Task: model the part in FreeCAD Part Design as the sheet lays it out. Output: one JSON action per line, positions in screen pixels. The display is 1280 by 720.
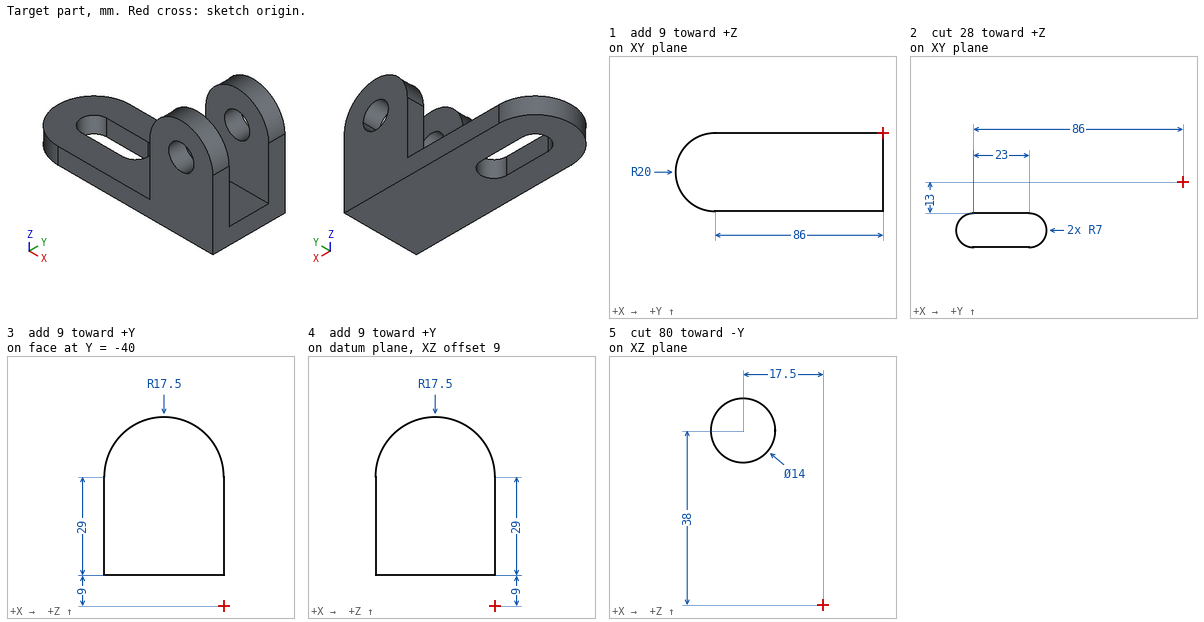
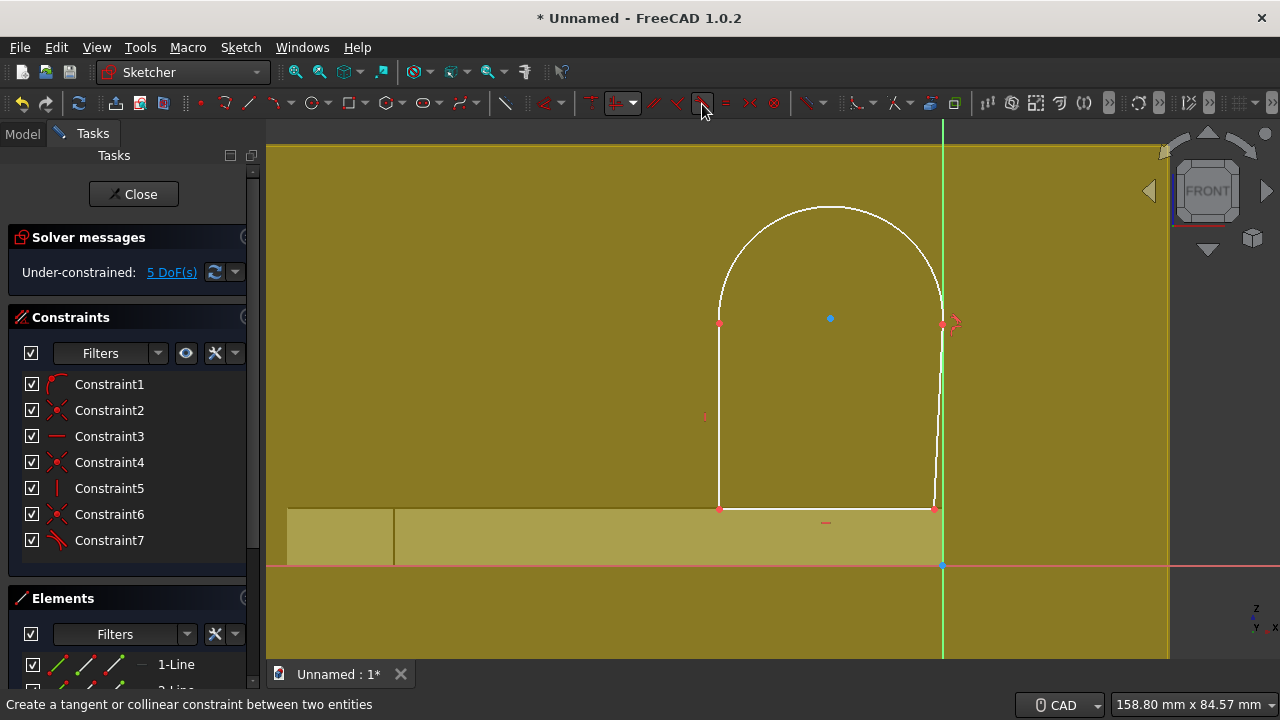
{"action": "left_click", "coordinate": [719, 454]}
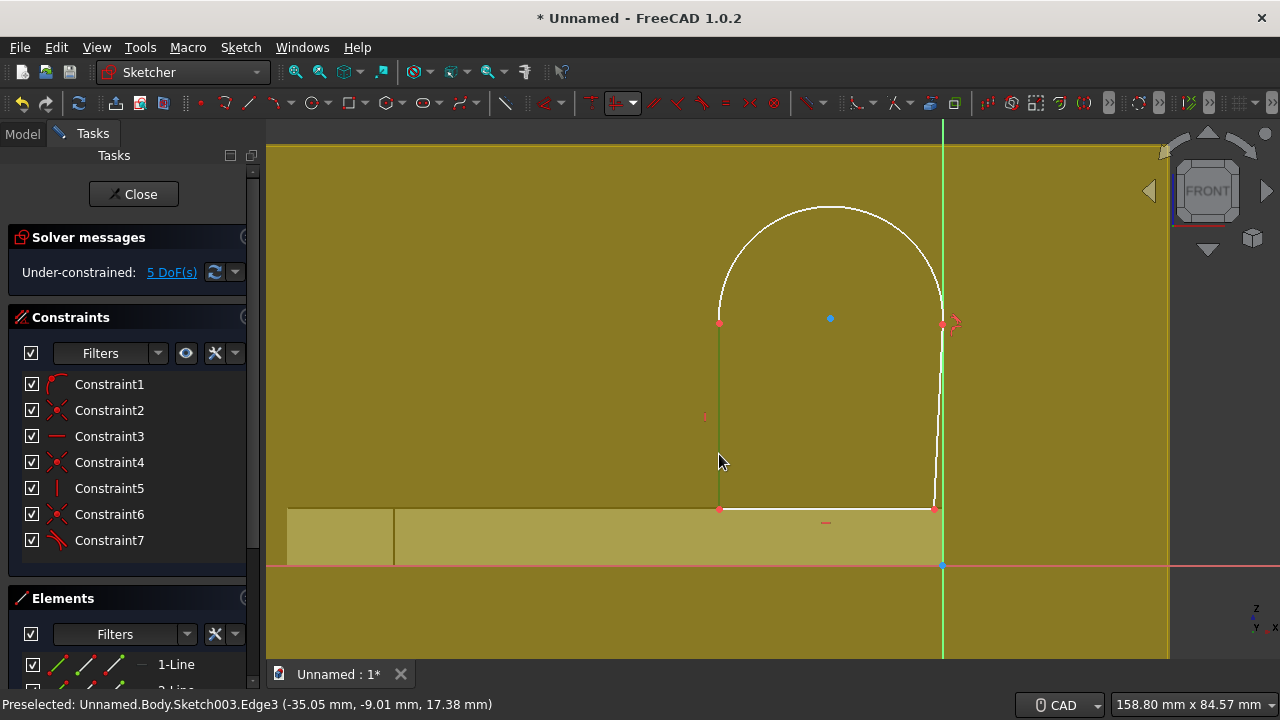
{"action": "left_click", "coordinate": [898, 229]}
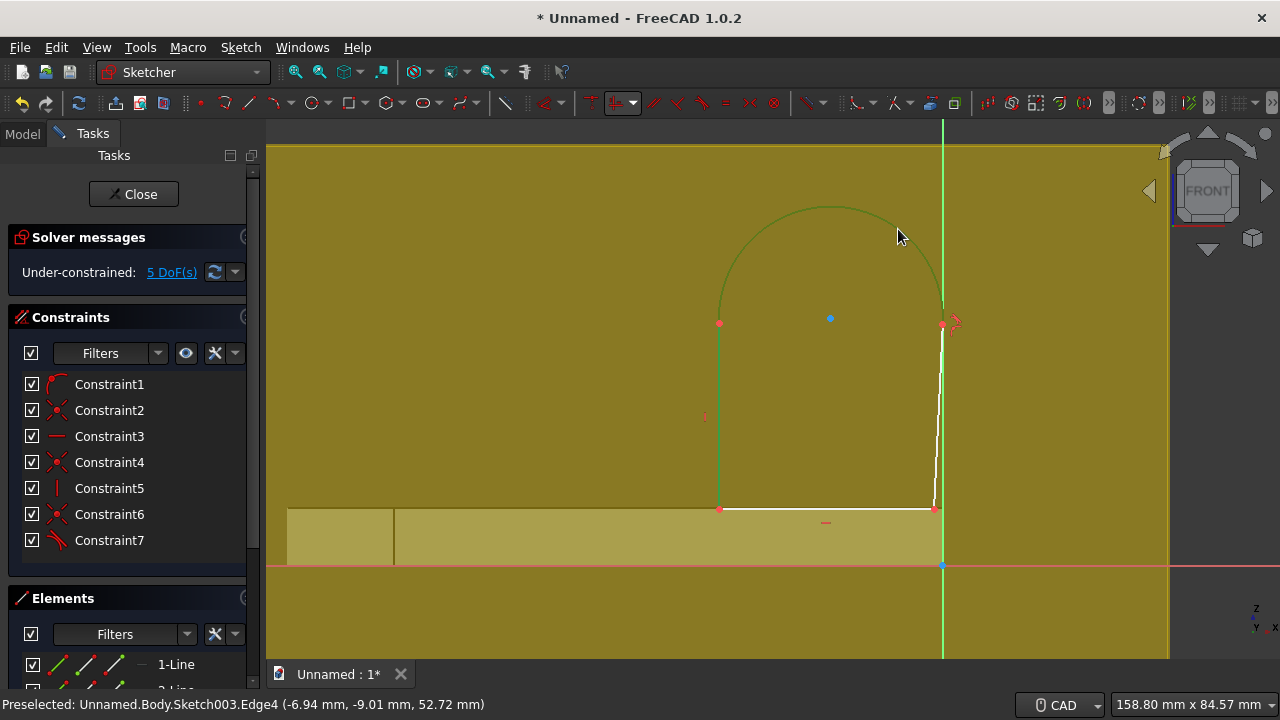
{"action": "left_click", "coordinate": [702, 104]}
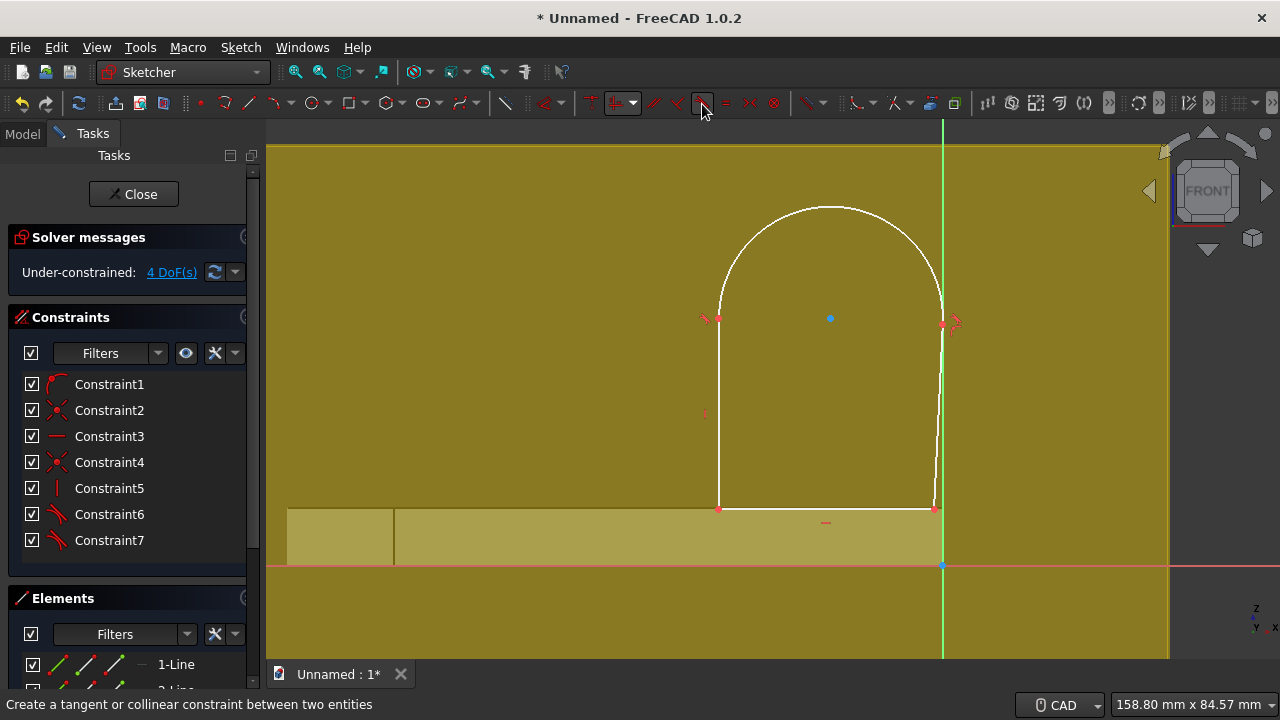
{"action": "left_click", "coordinate": [940, 380]}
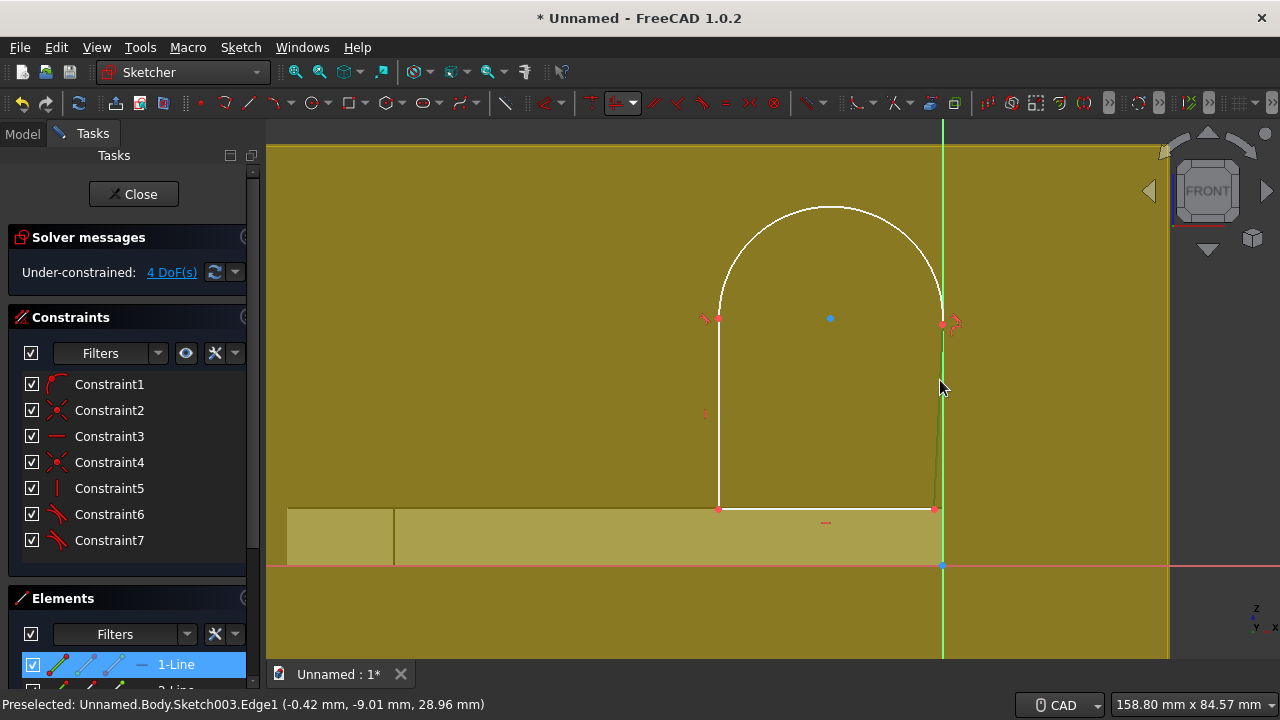
{"action": "left_click", "coordinate": [636, 104]}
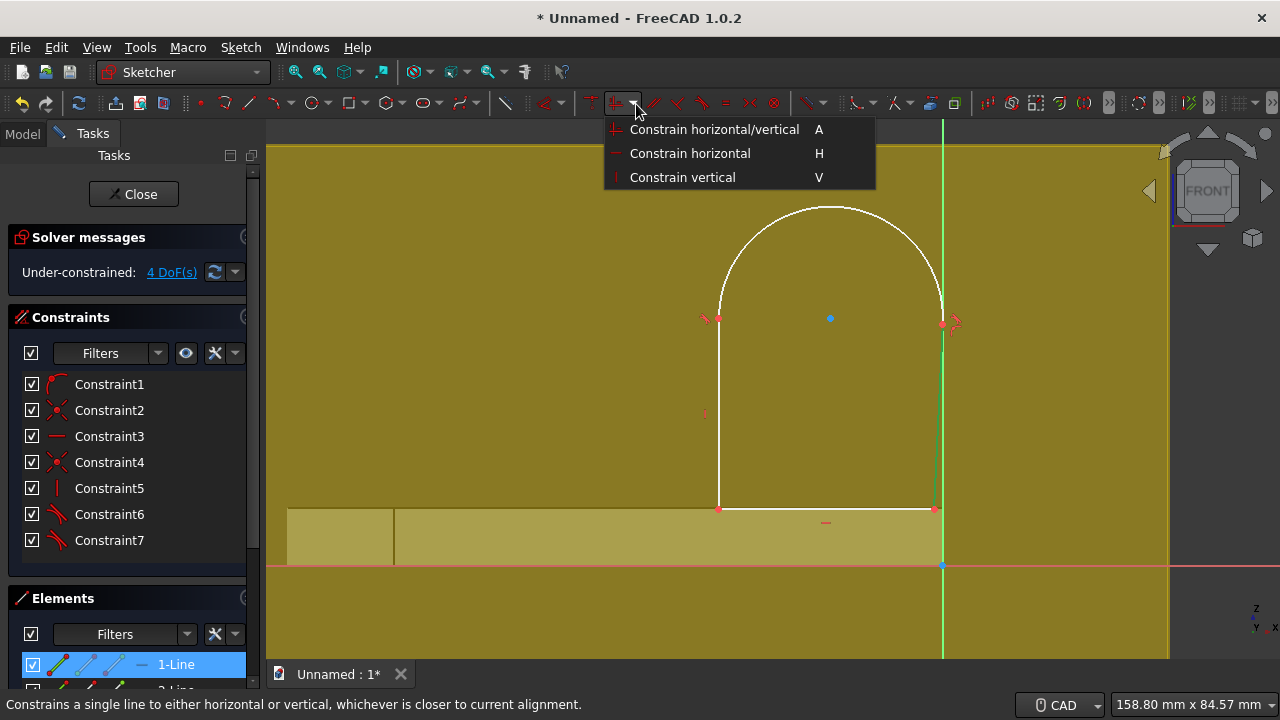
{"action": "left_click", "coordinate": [740, 177]}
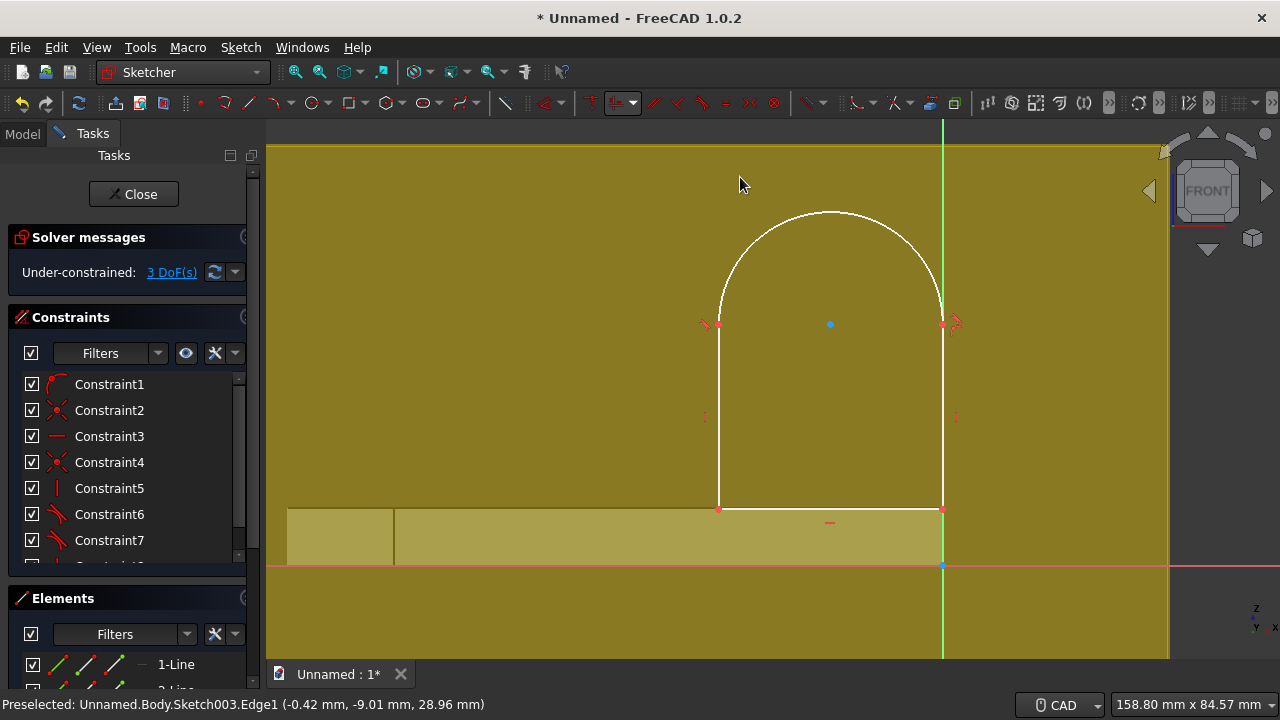
{"action": "left_click", "coordinate": [544, 104]}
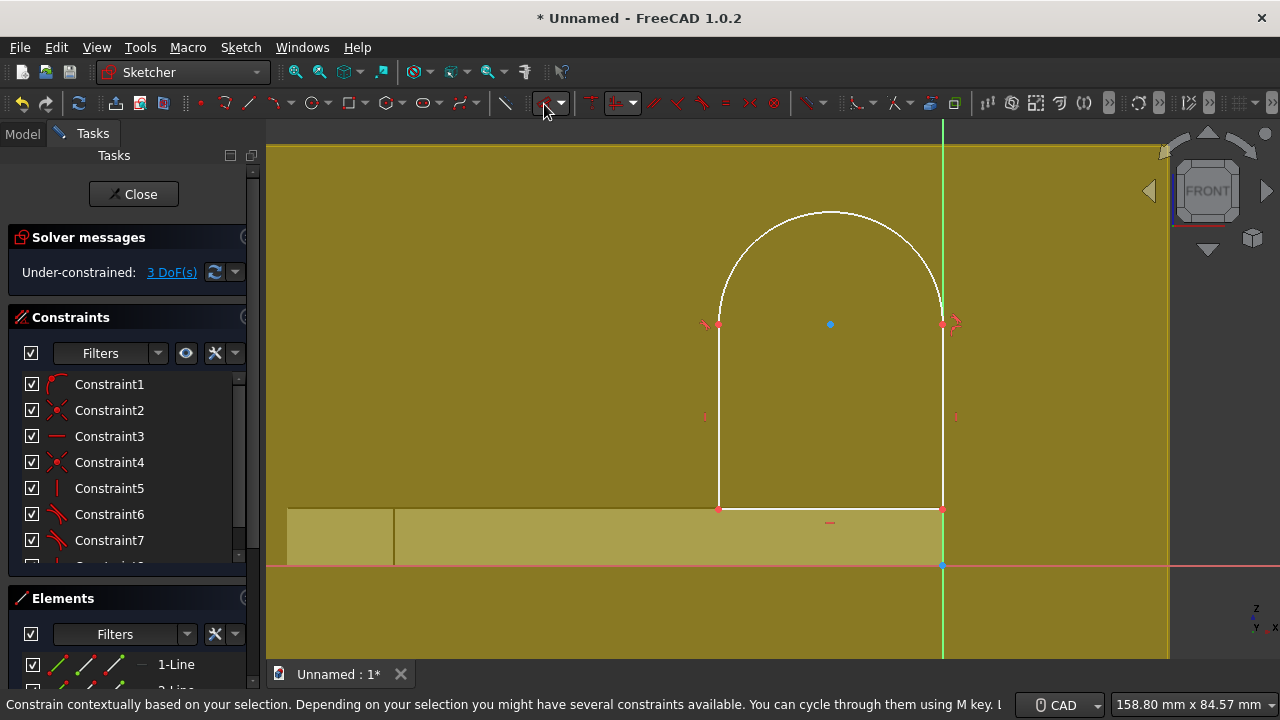
{"action": "left_click", "coordinate": [897, 233]}
{"action": "left_click", "coordinate": [916, 207]}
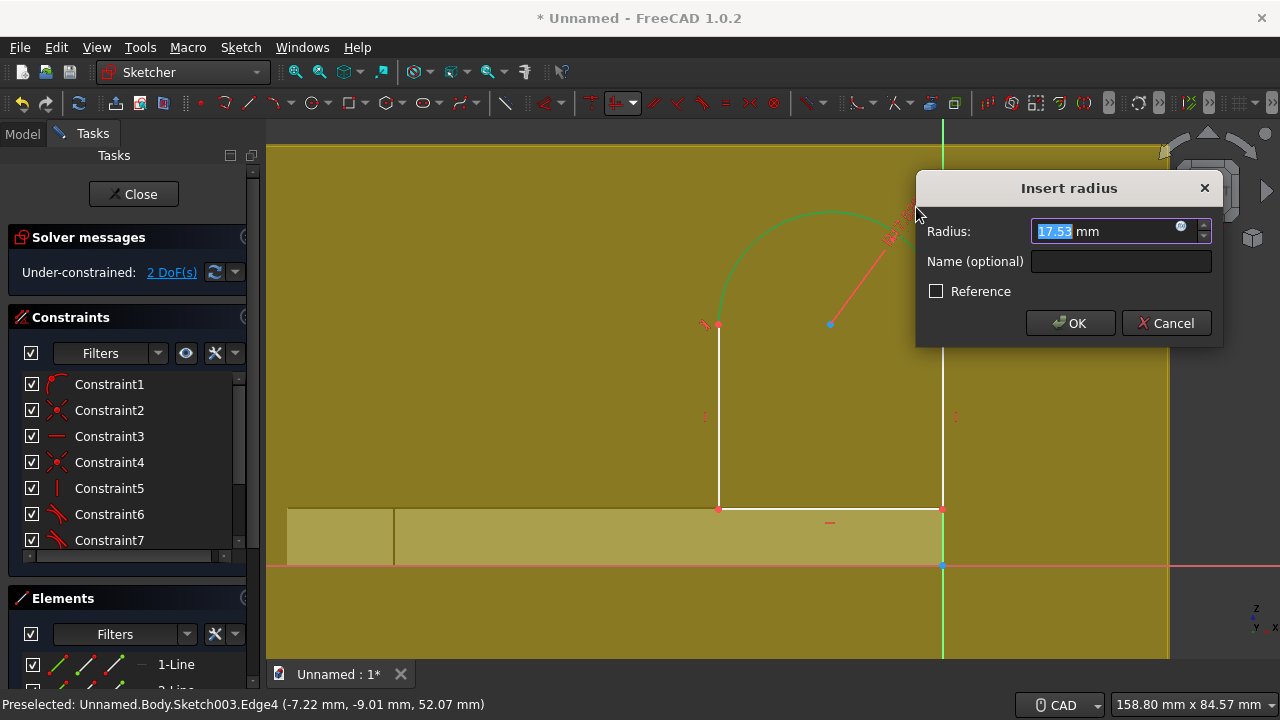
{"action": "type", "text": "17.5"}
{"action": "key", "text": "Return"}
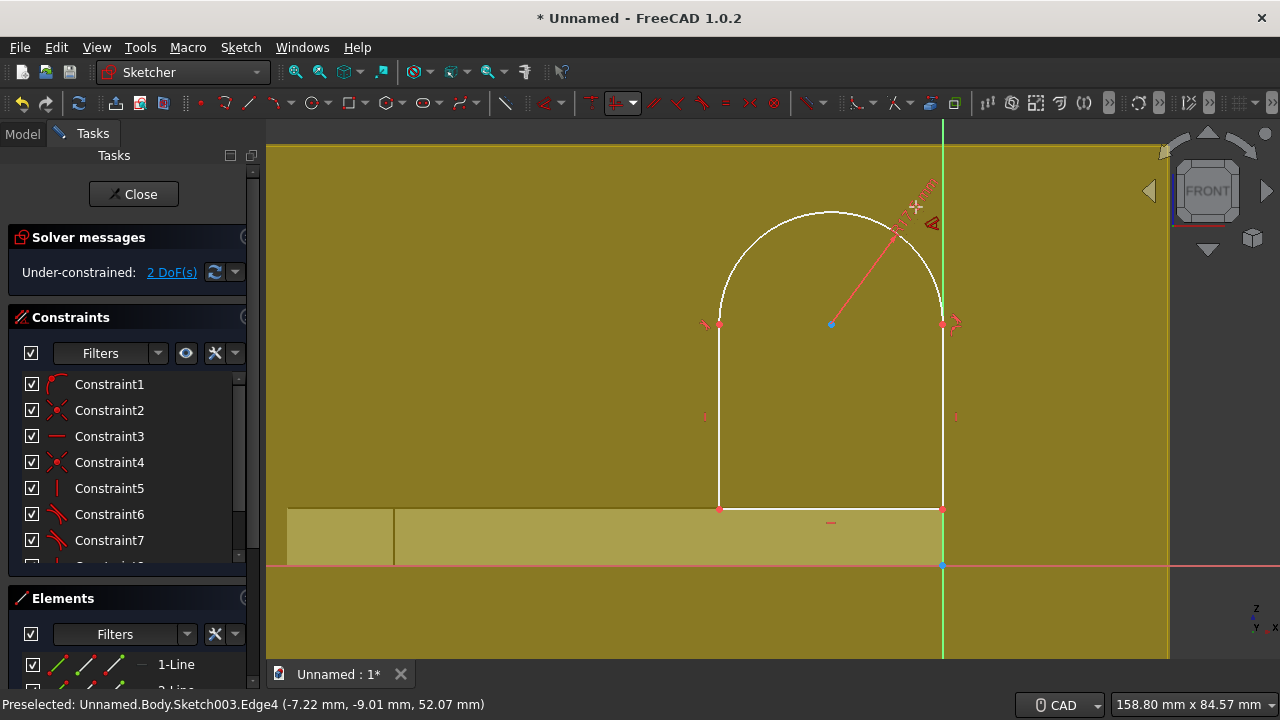
{"action": "left_click", "coordinate": [943, 380]}
{"action": "left_click", "coordinate": [977, 417]}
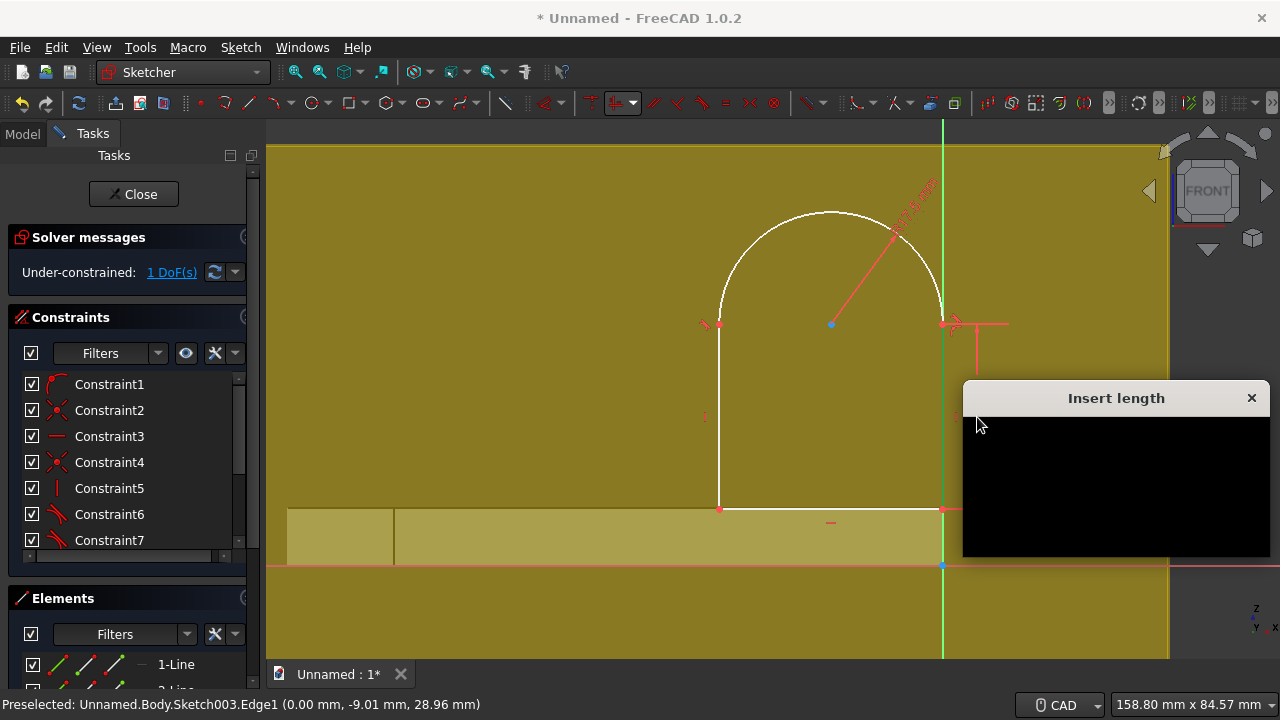
{"action": "type", "text": "29"}
{"action": "key", "text": "Return"}